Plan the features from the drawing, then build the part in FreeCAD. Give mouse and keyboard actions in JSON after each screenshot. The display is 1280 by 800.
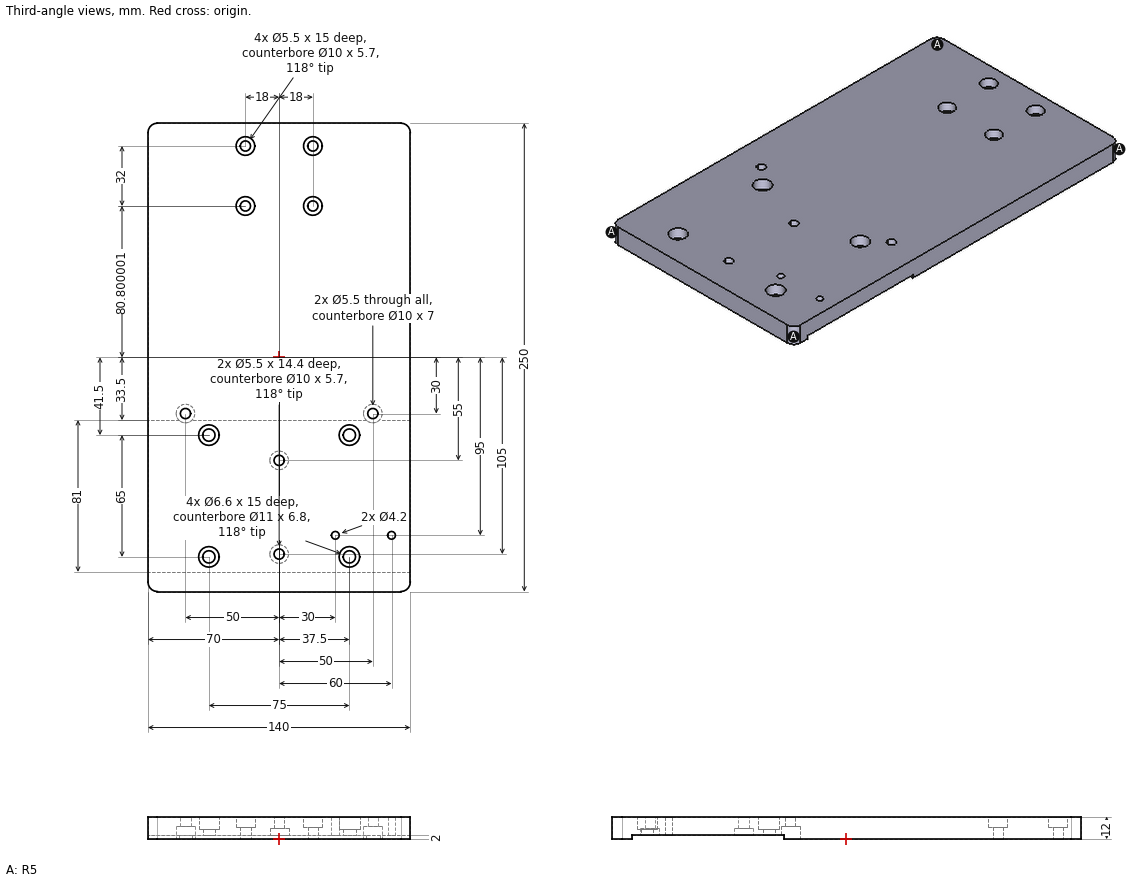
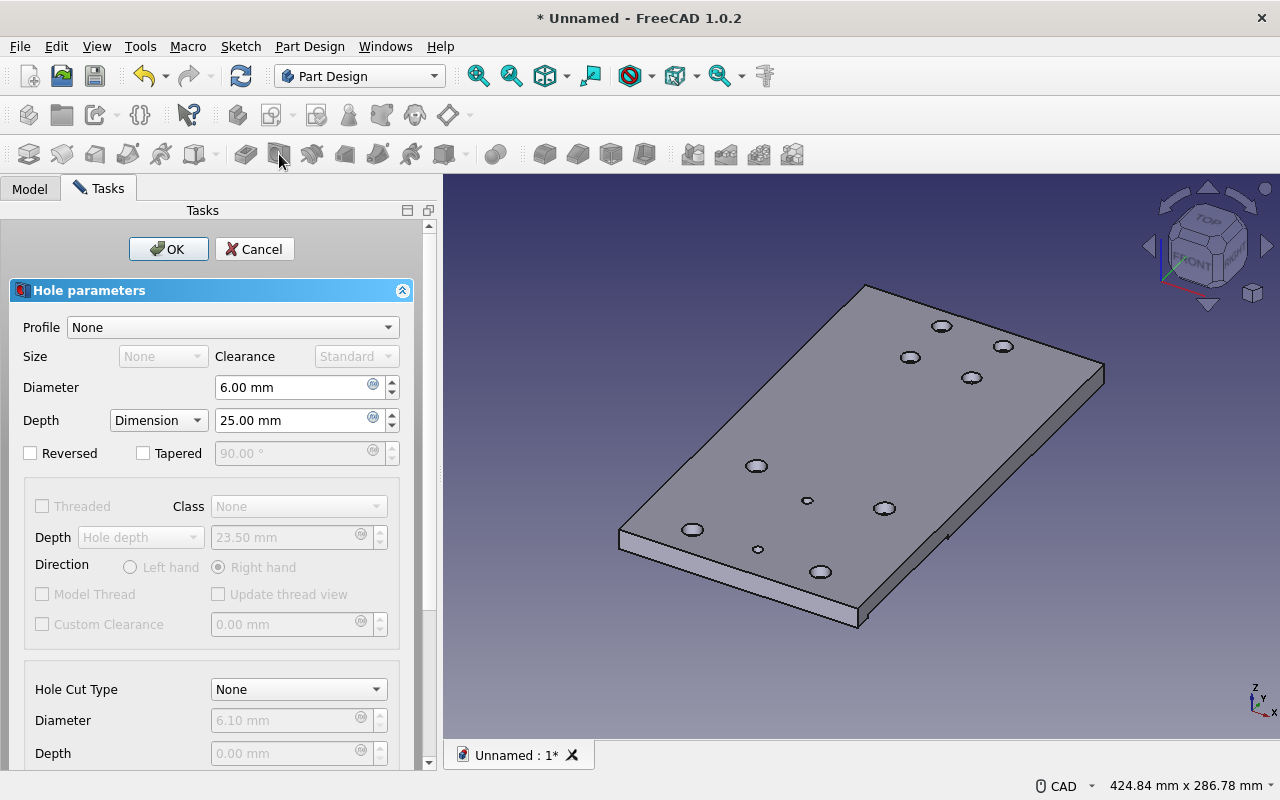
{"action": "triple_click", "coordinate": [300, 388]}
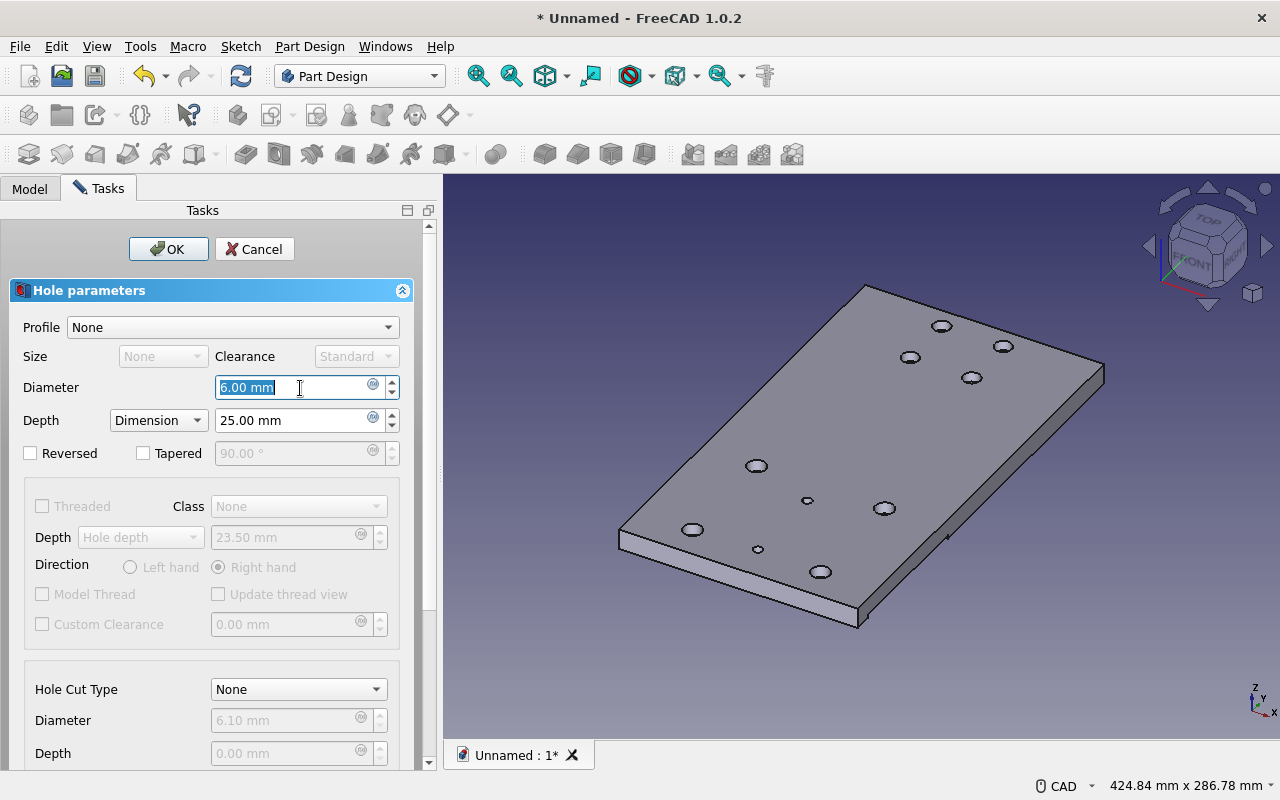
{"action": "type", "text": "5.5"}
{"action": "key", "text": "Tab"}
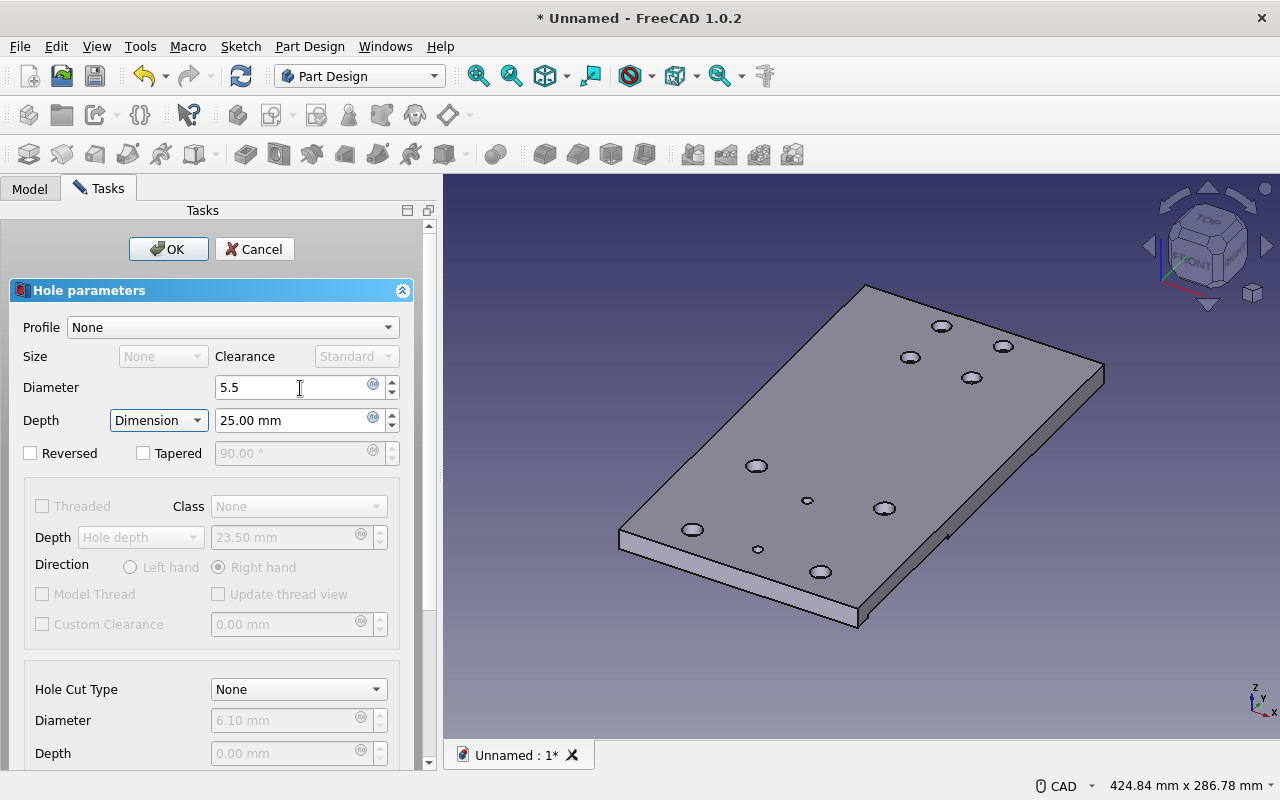
{"action": "left_click", "coordinate": [160, 420]}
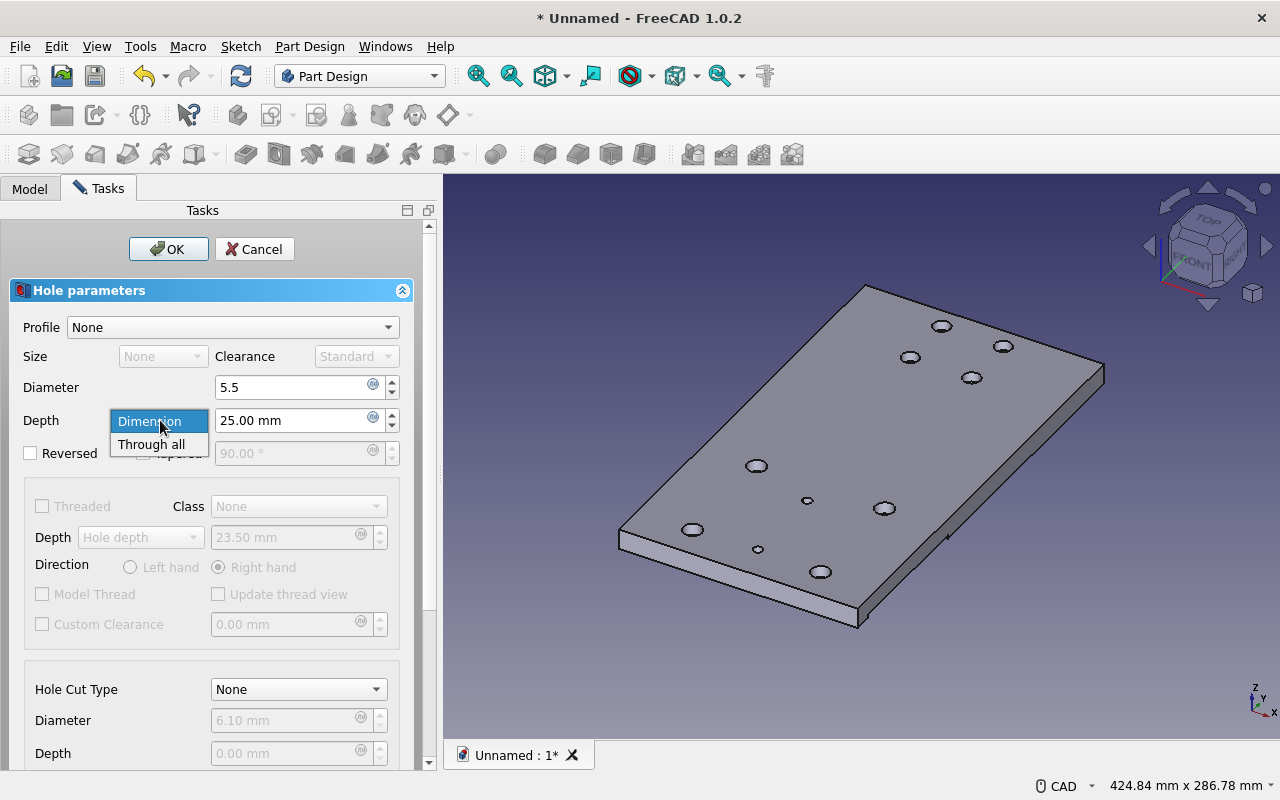
{"action": "left_click", "coordinate": [158, 444]}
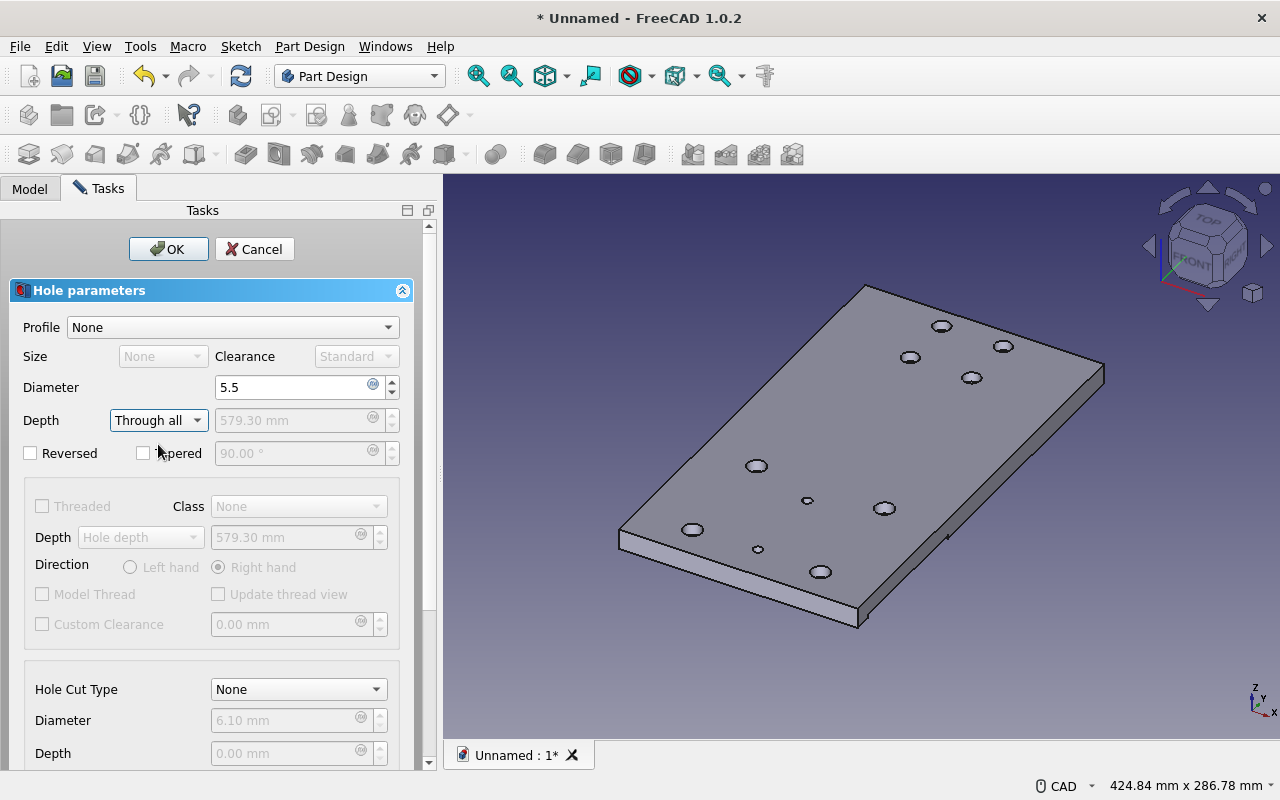
{"action": "left_click", "coordinate": [31, 453]}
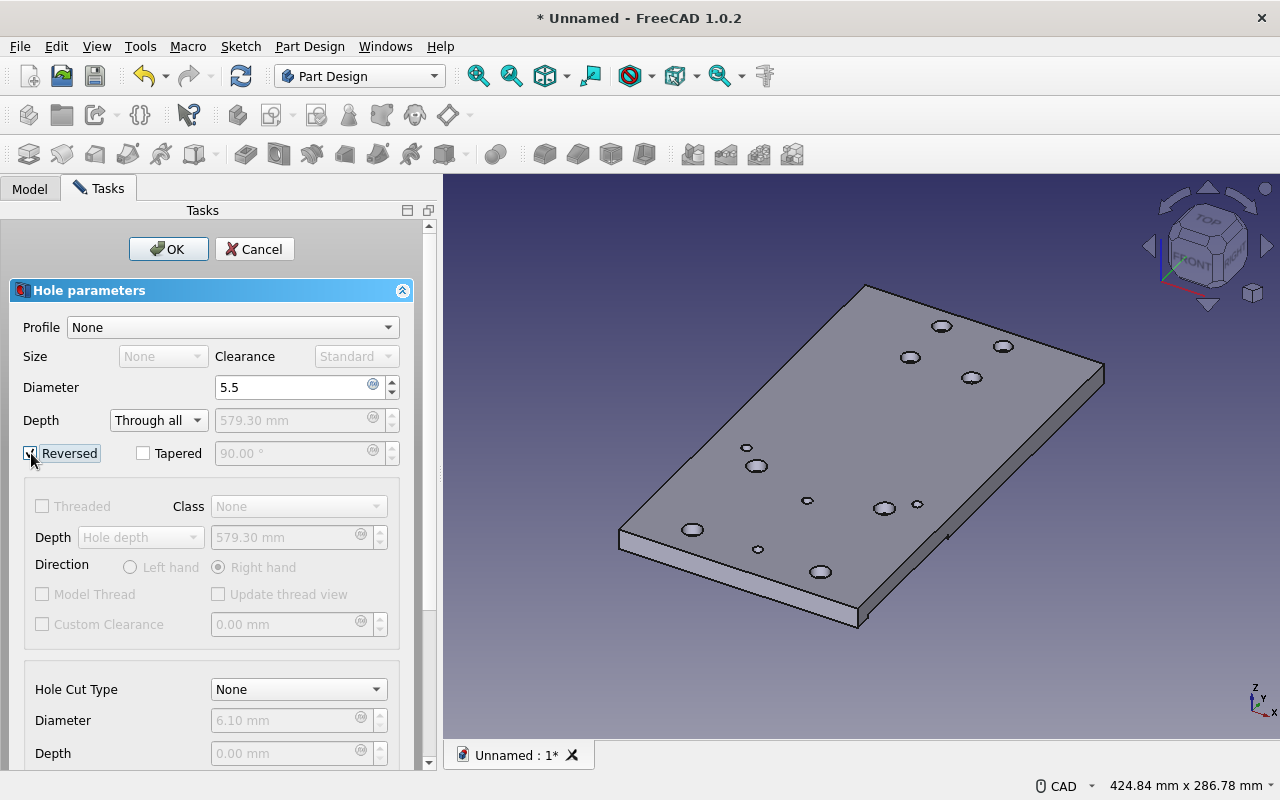
{"action": "left_click", "coordinate": [300, 690]}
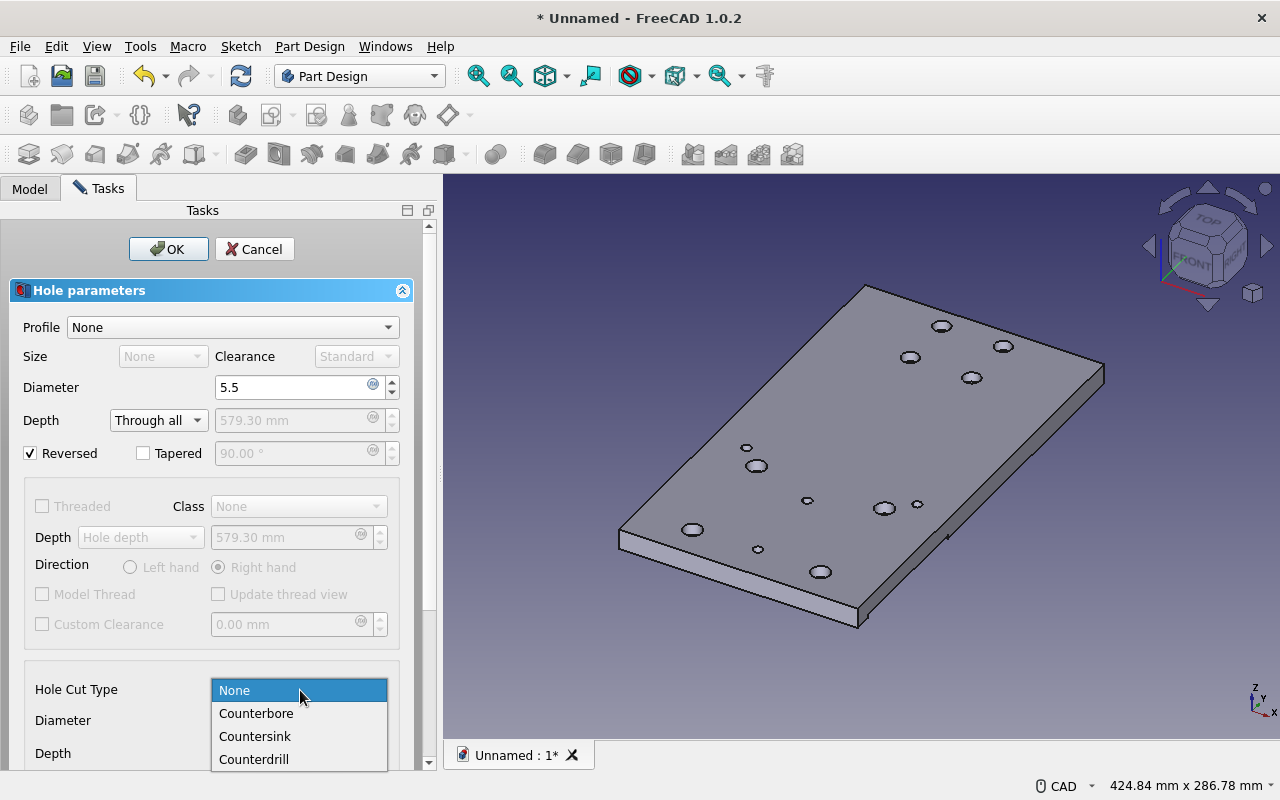
{"action": "left_click", "coordinate": [298, 714]}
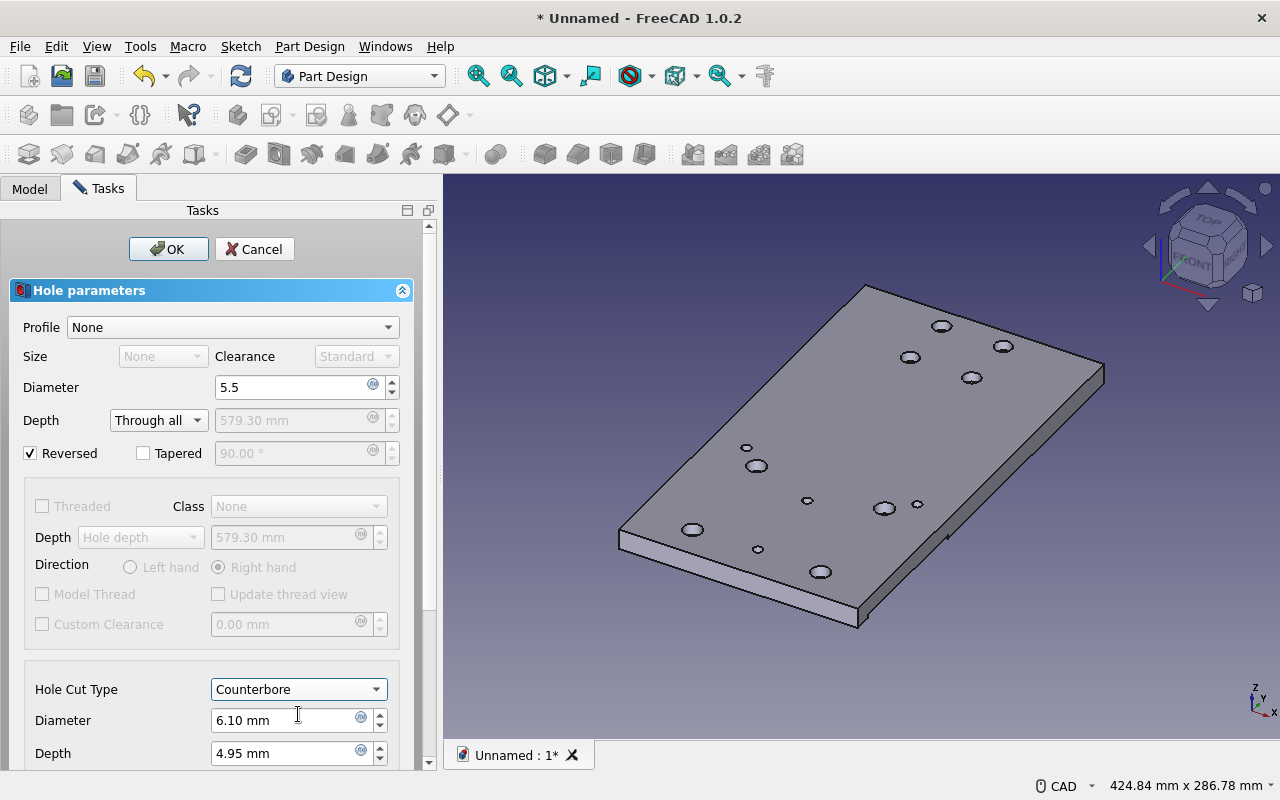
{"action": "triple_click", "coordinate": [292, 720]}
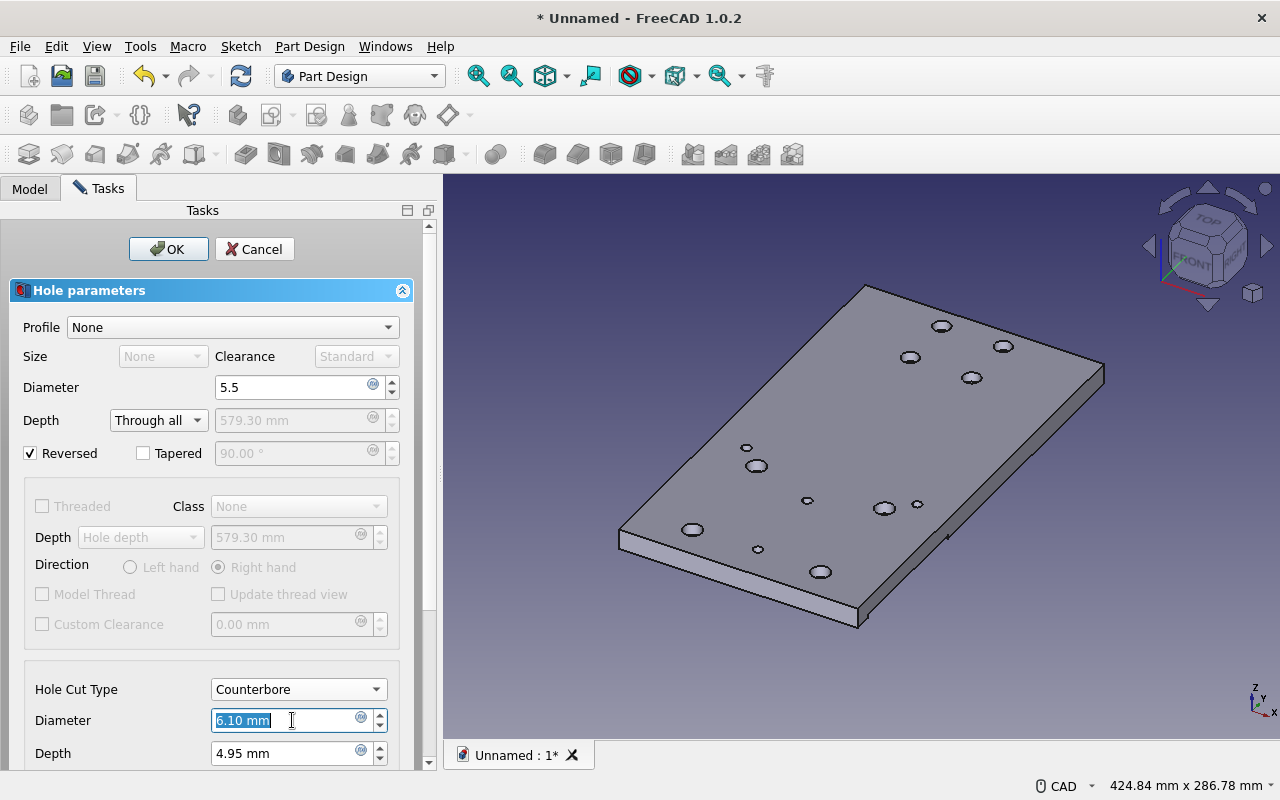
{"action": "type", "text": "10"}
{"action": "key", "text": "Tab"}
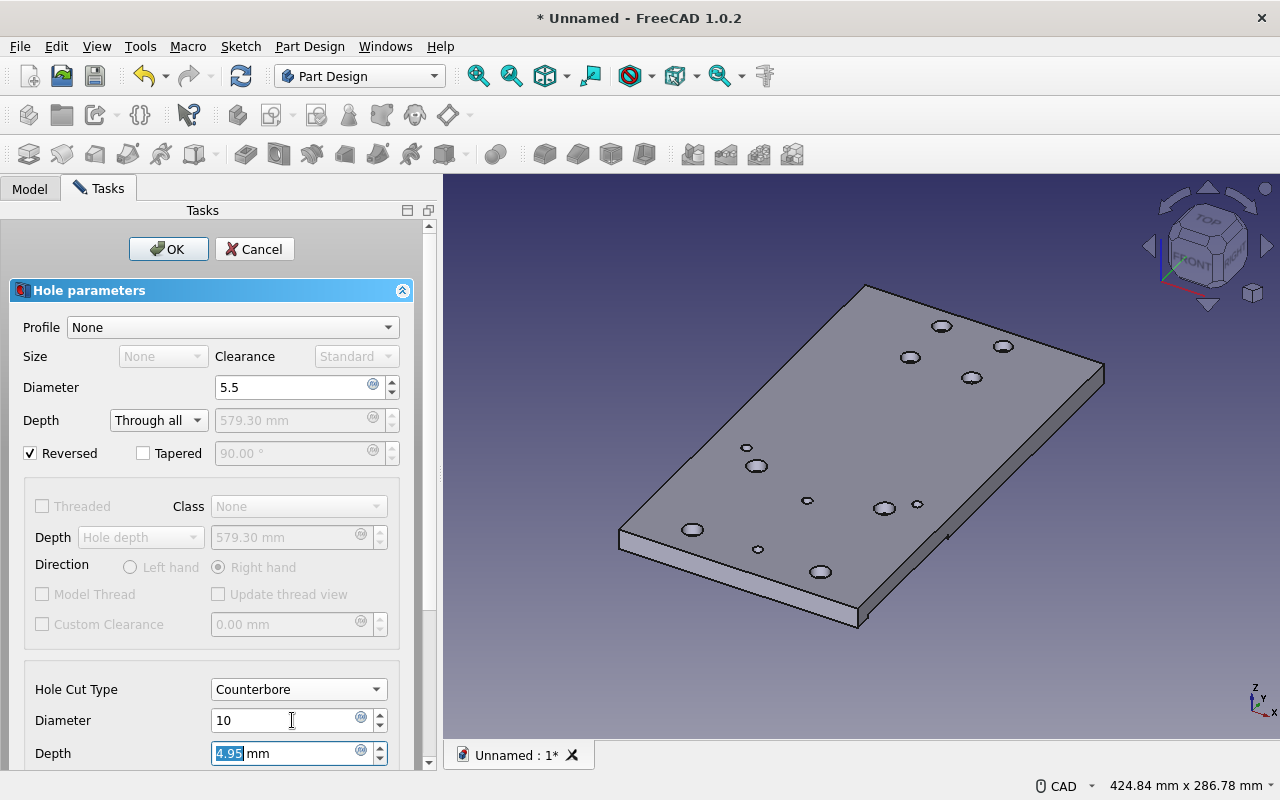
{"action": "type", "text": "7"}
{"action": "key", "text": "Tab"}